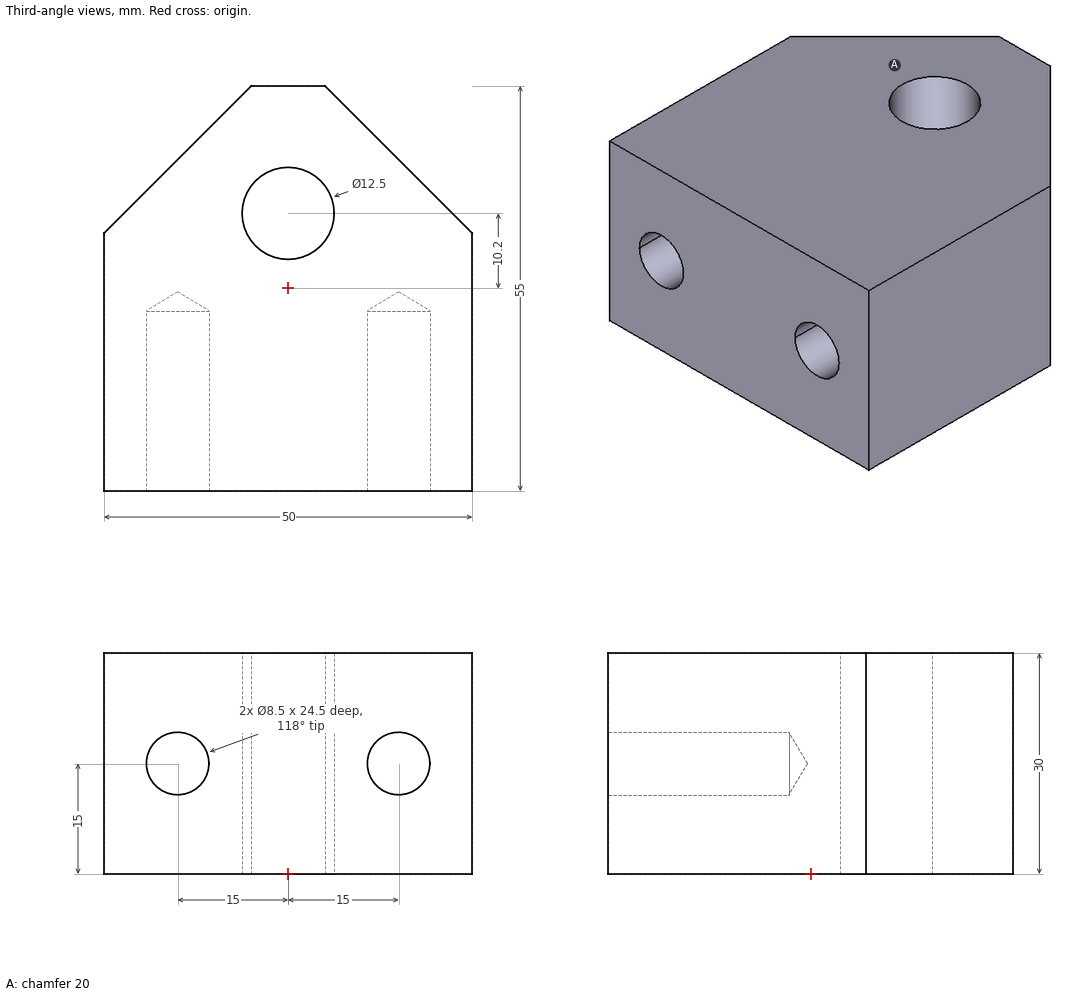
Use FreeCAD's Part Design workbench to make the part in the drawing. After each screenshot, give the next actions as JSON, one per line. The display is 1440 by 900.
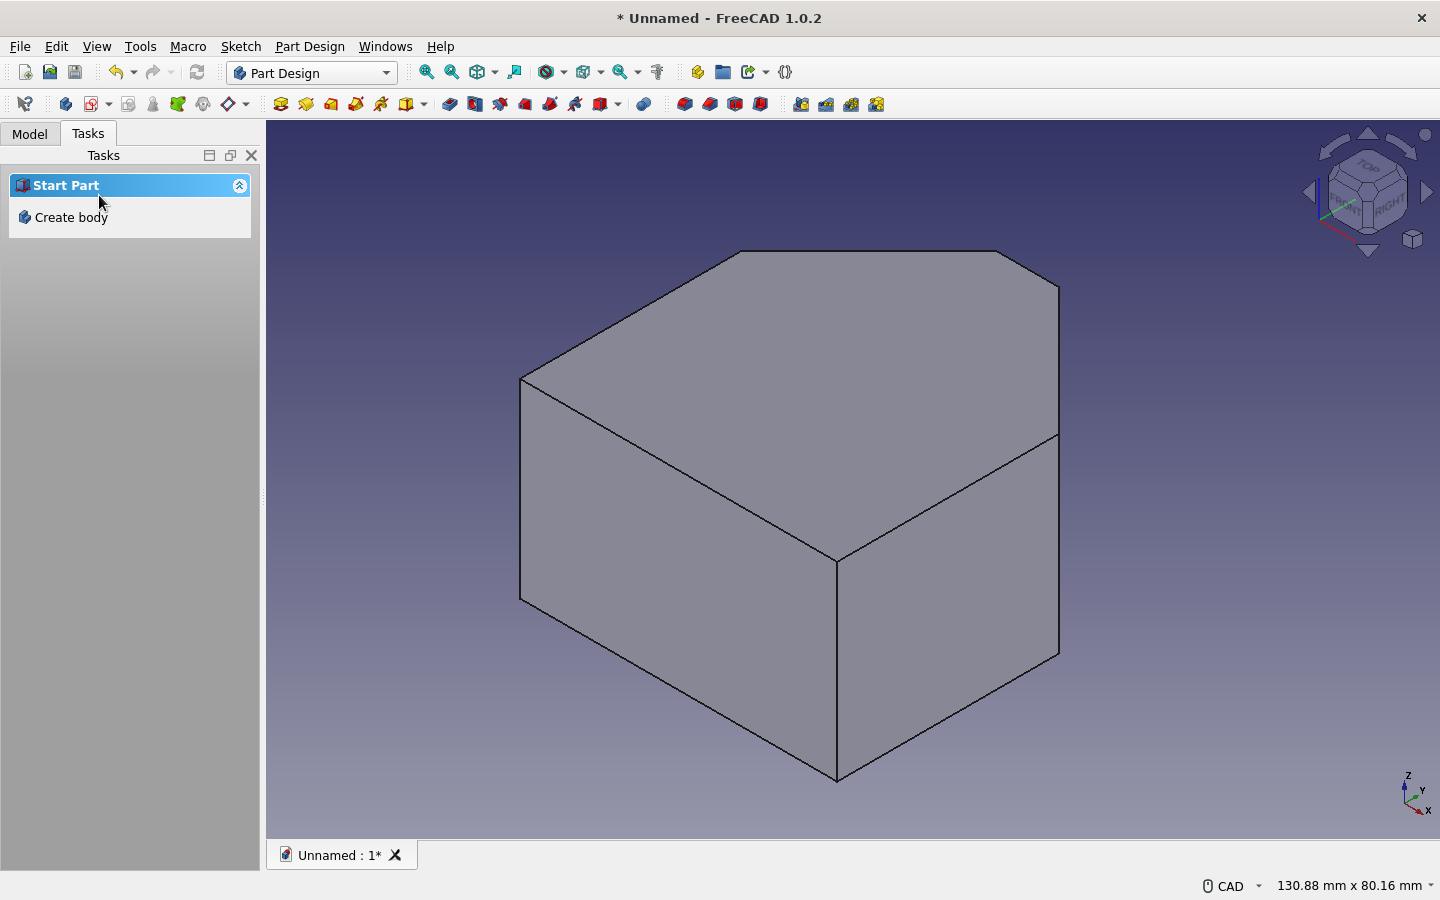
{"action": "left_click", "coordinate": [724, 605]}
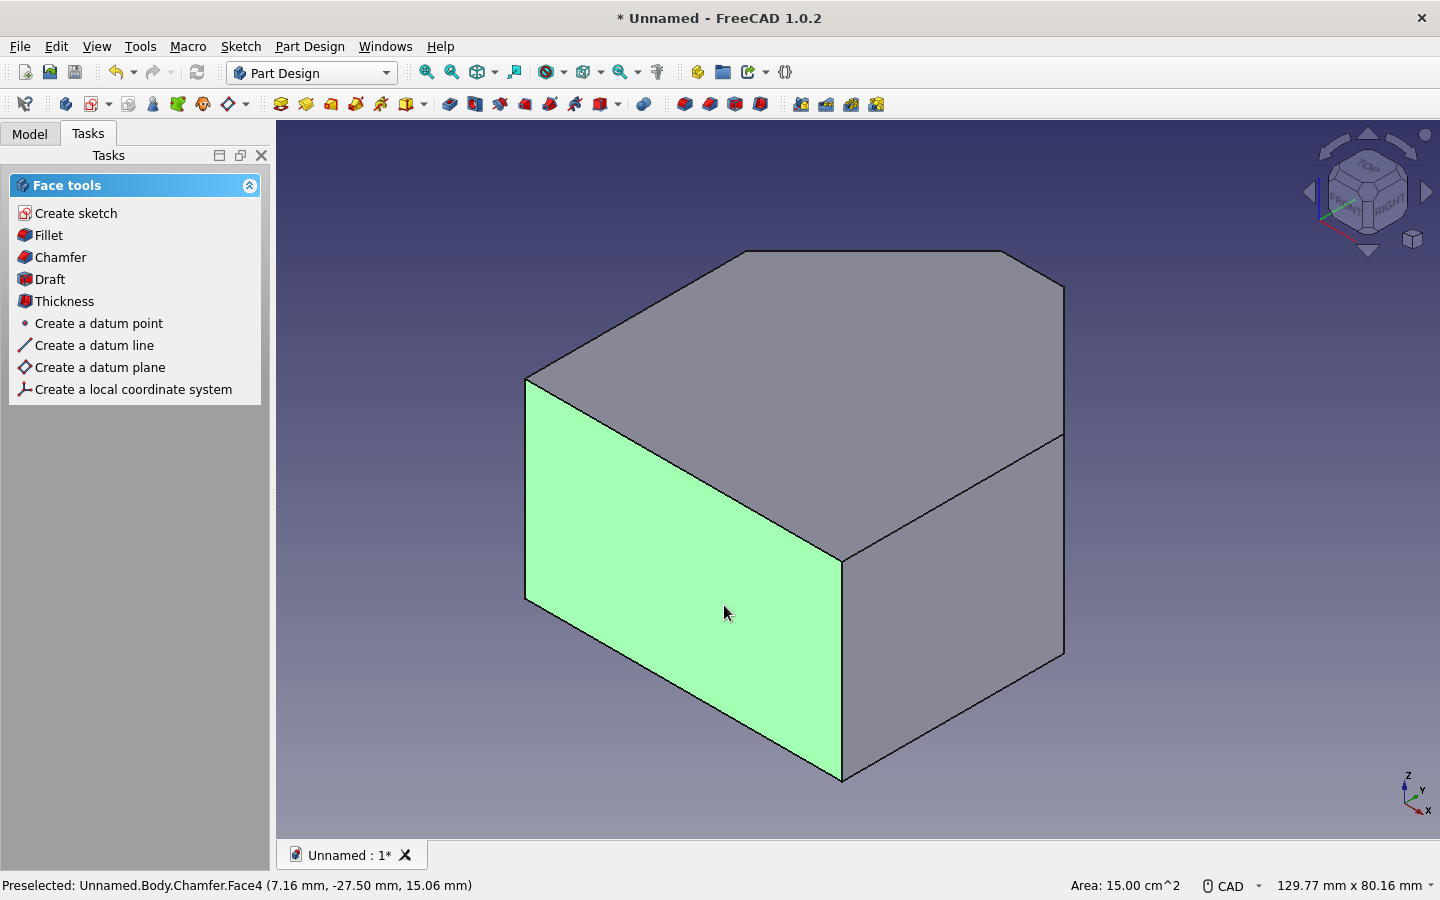
{"action": "left_click", "coordinate": [90, 104]}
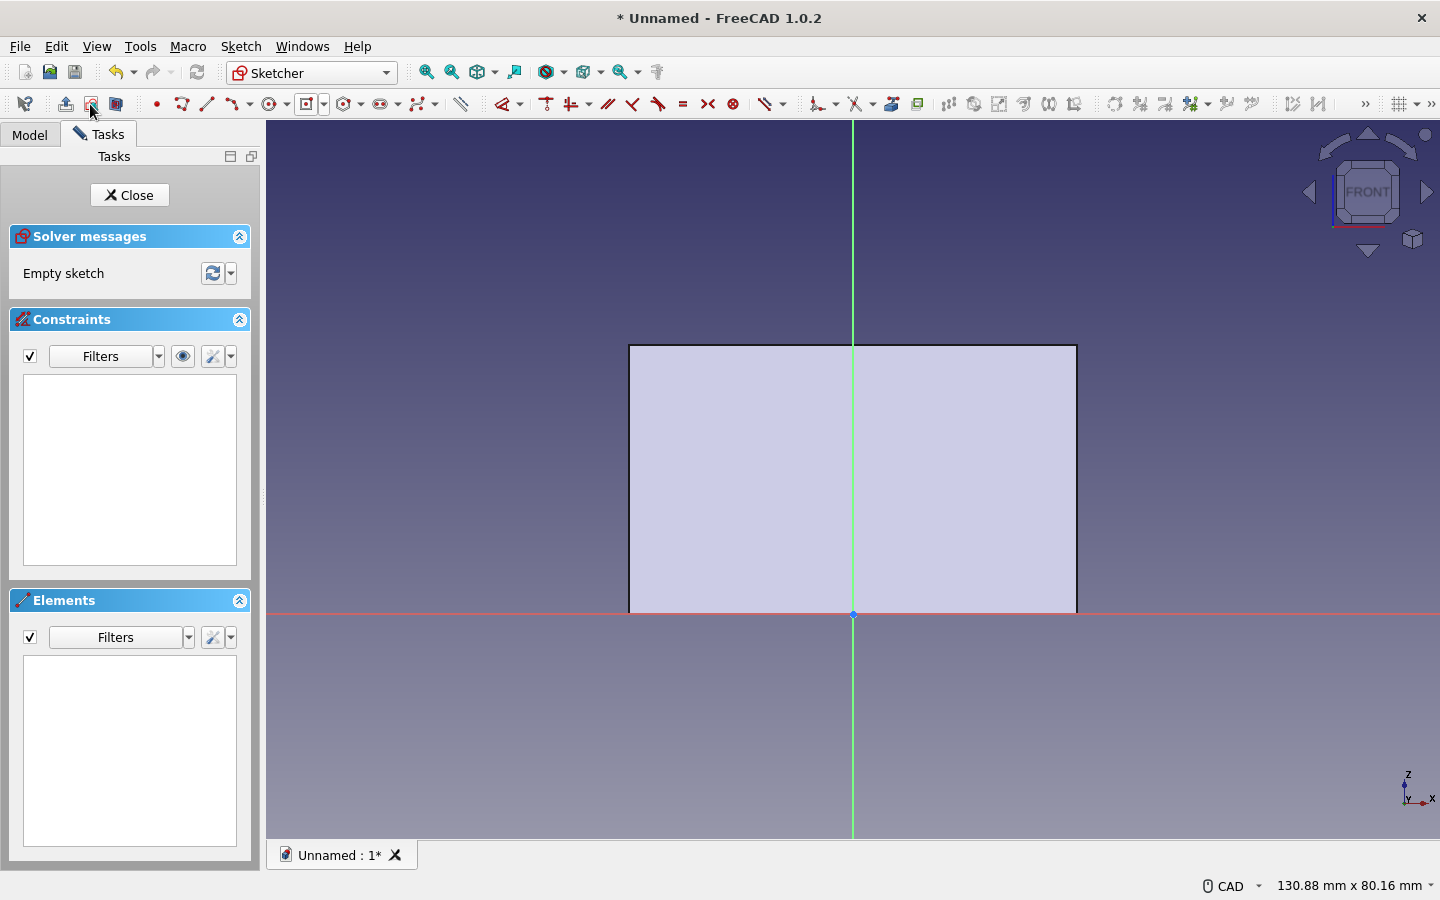
{"action": "scroll", "coordinate": [936, 586], "scroll_direction": "up", "scroll_amount": 3}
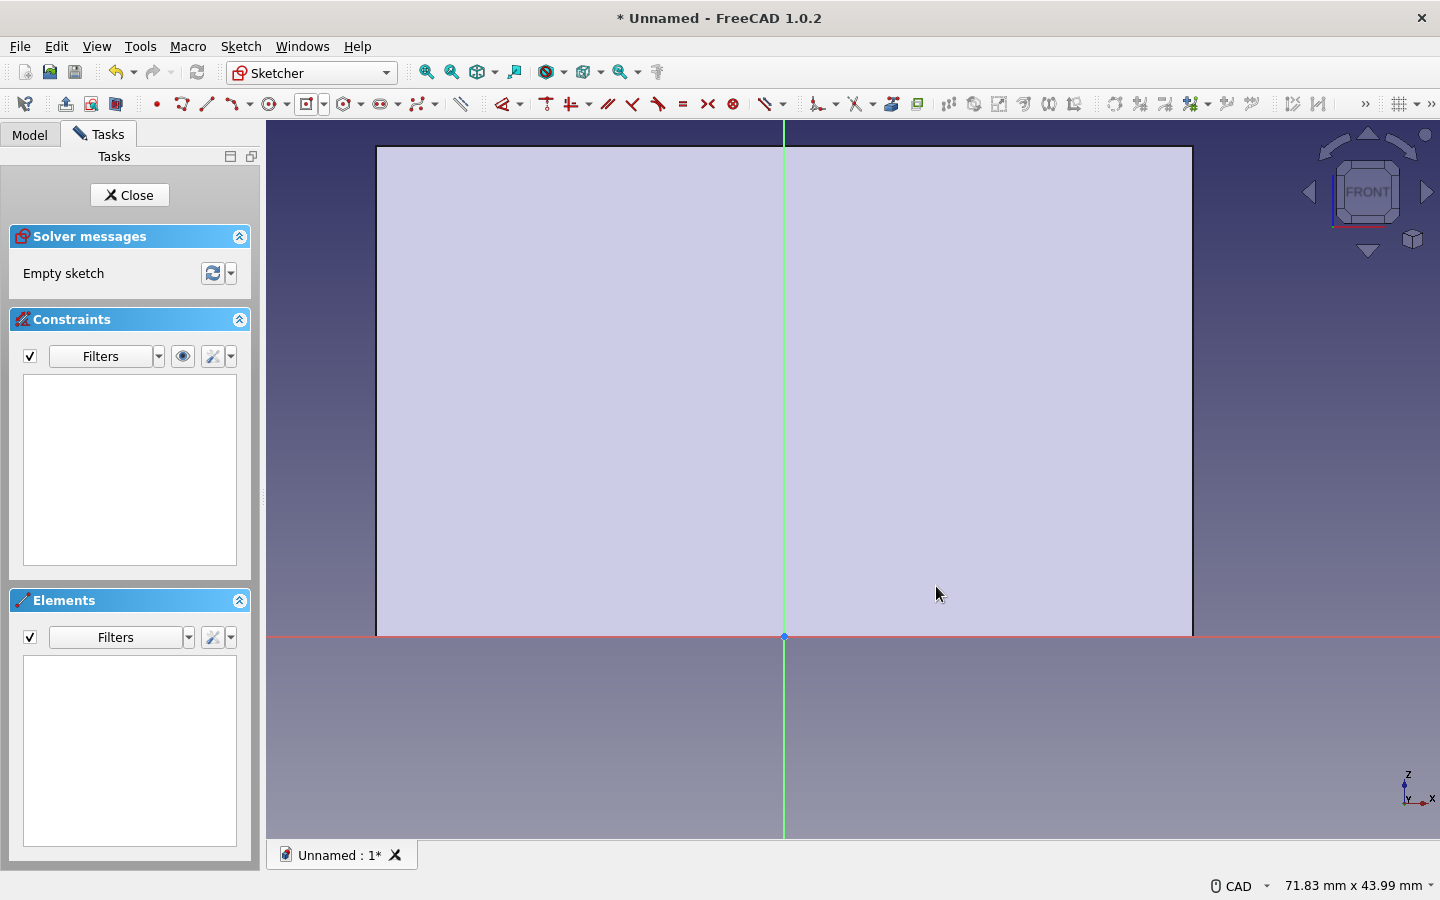
{"action": "left_click", "coordinate": [268, 104]}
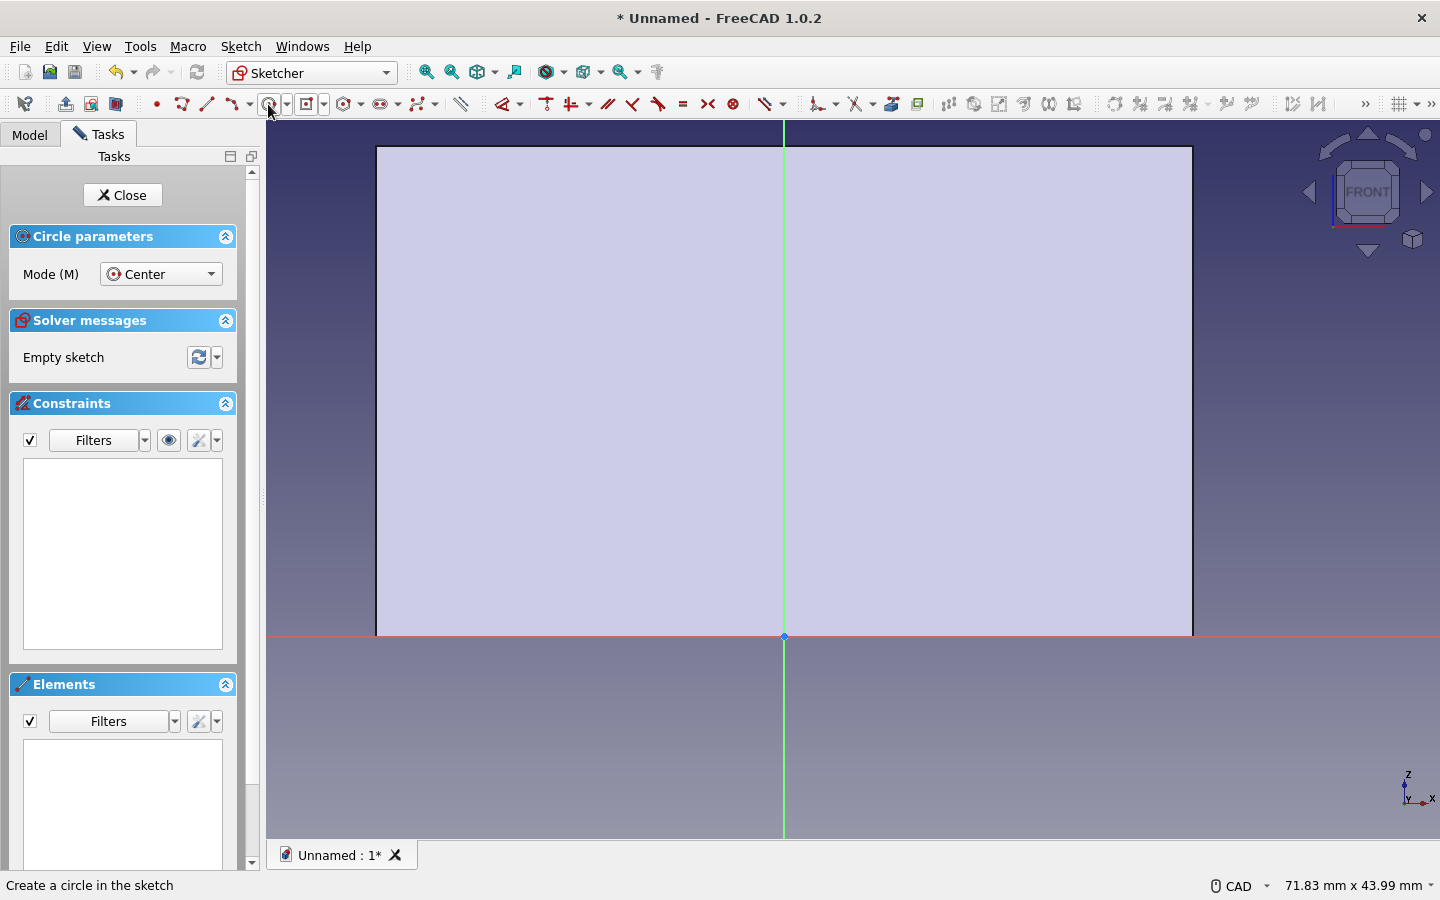
{"action": "left_click", "coordinate": [539, 391]}
{"action": "mouse_move", "coordinate": [588, 342]}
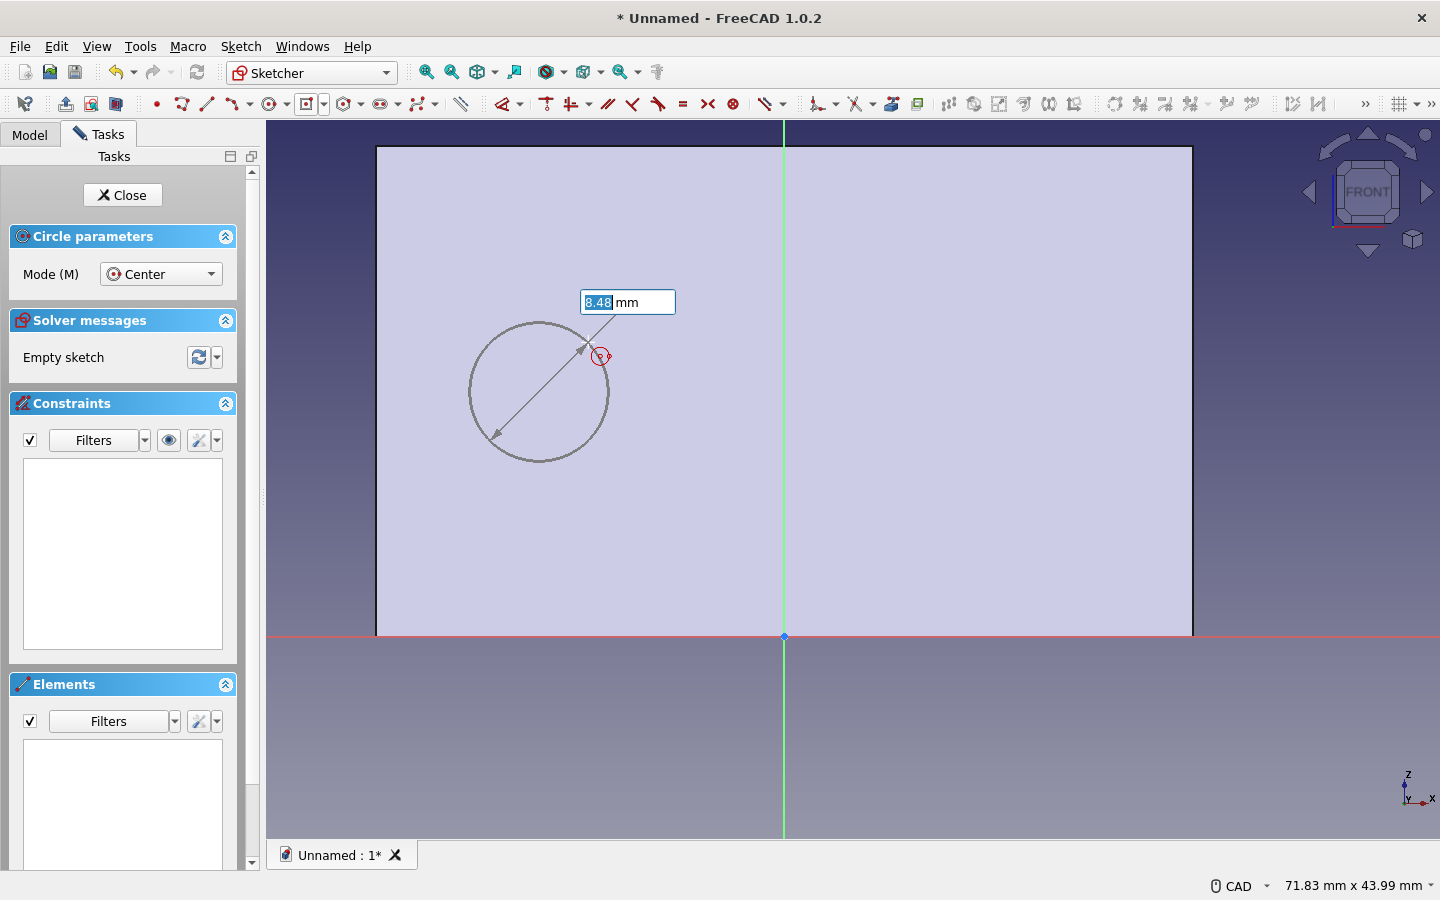
{"action": "type", "text": "8.5"}
{"action": "key", "text": "Return"}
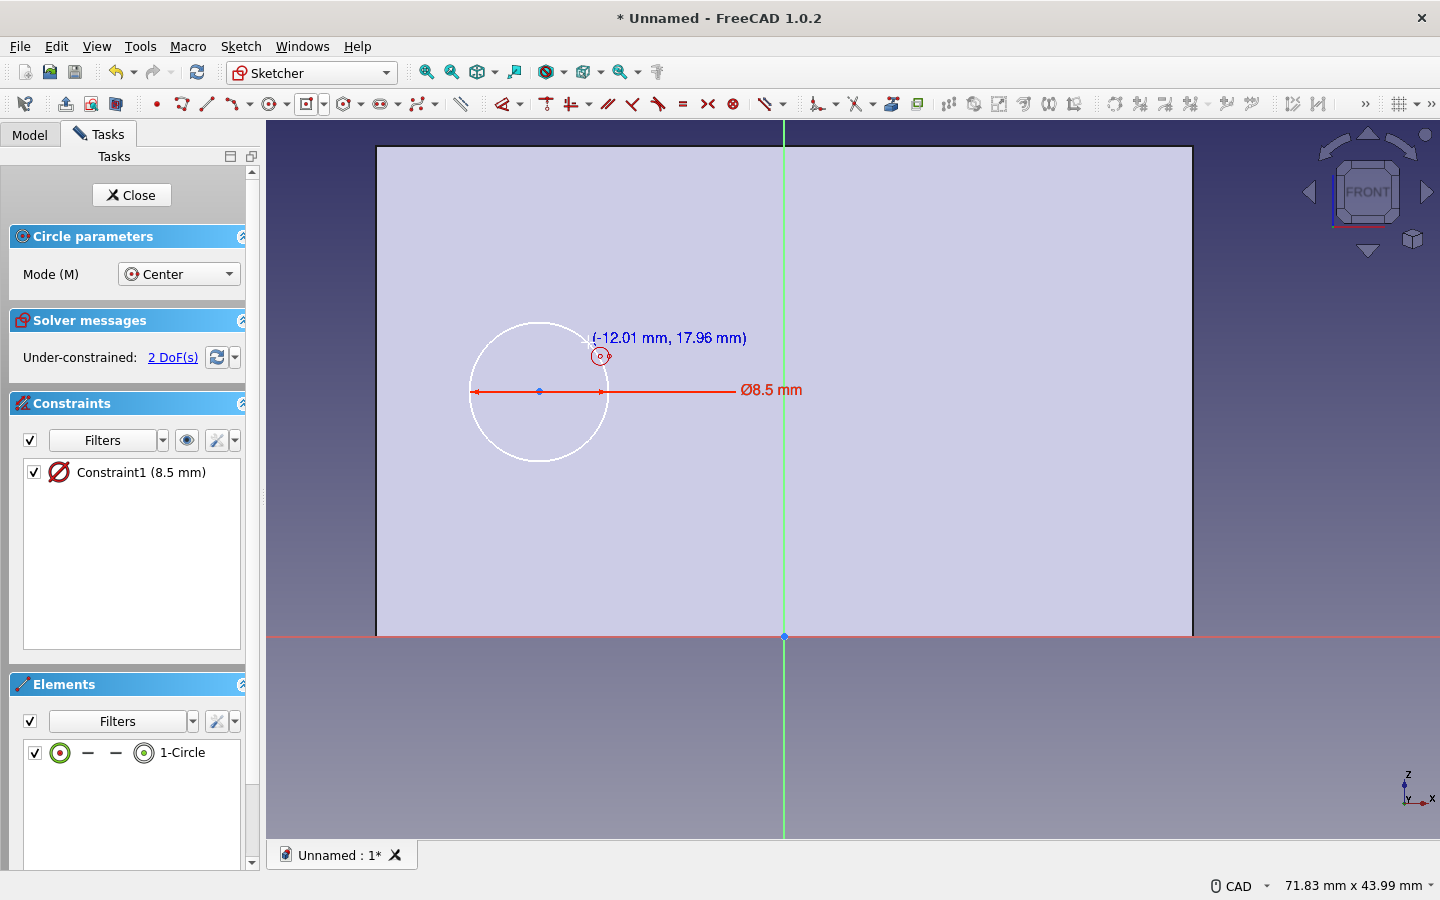
{"action": "left_click", "coordinate": [1029, 391]}
{"action": "mouse_move", "coordinate": [1079, 342]}